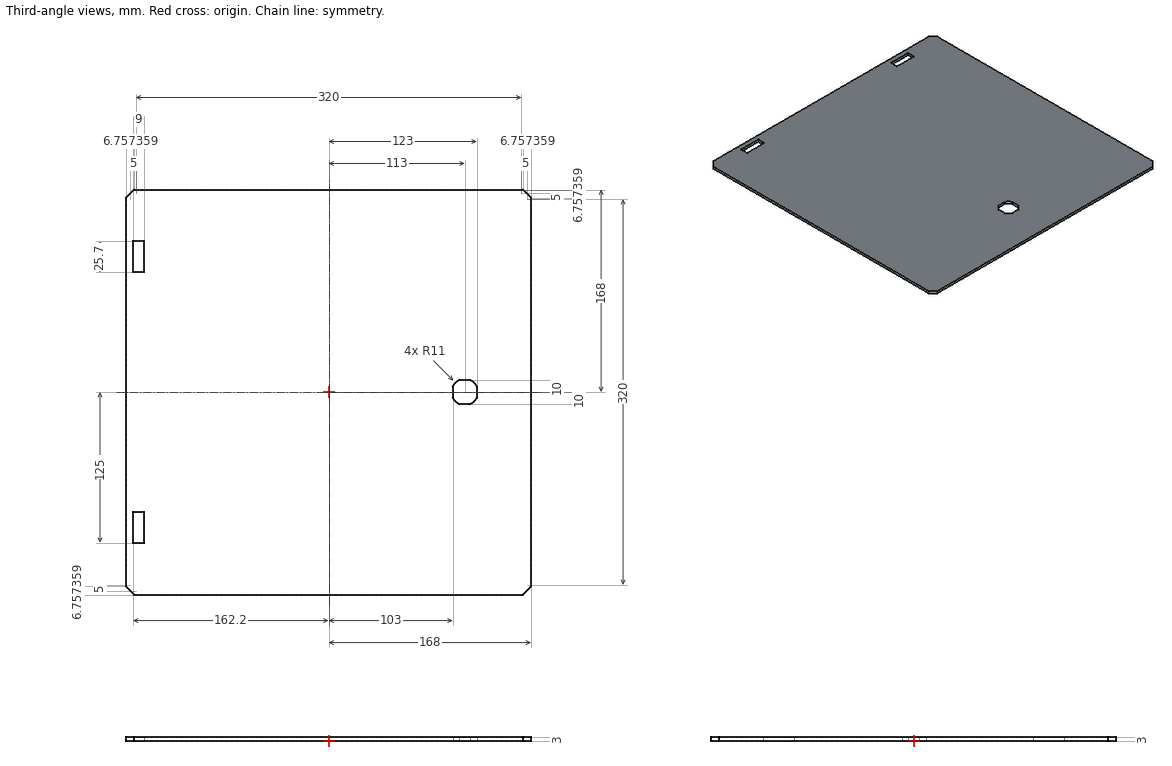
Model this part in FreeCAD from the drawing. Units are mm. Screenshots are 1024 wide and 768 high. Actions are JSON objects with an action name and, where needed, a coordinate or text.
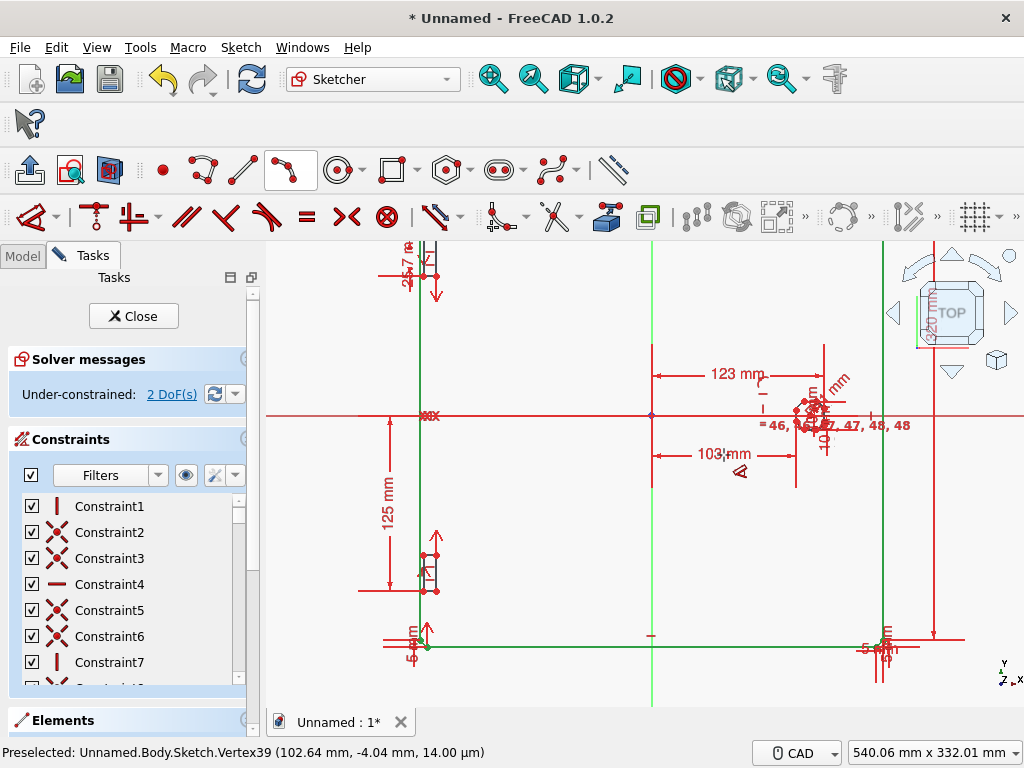
{"action": "left_click", "coordinate": [811, 416]}
{"action": "left_click", "coordinate": [731, 498]}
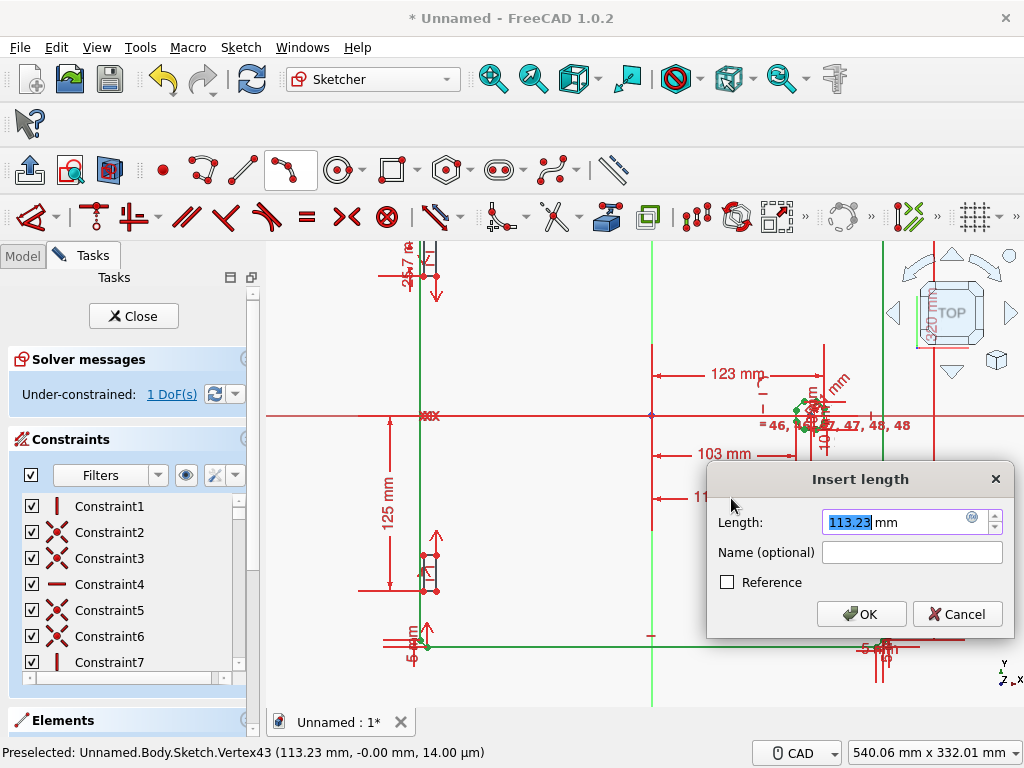
{"action": "type", "text": "113"}
{"action": "key", "text": "Return"}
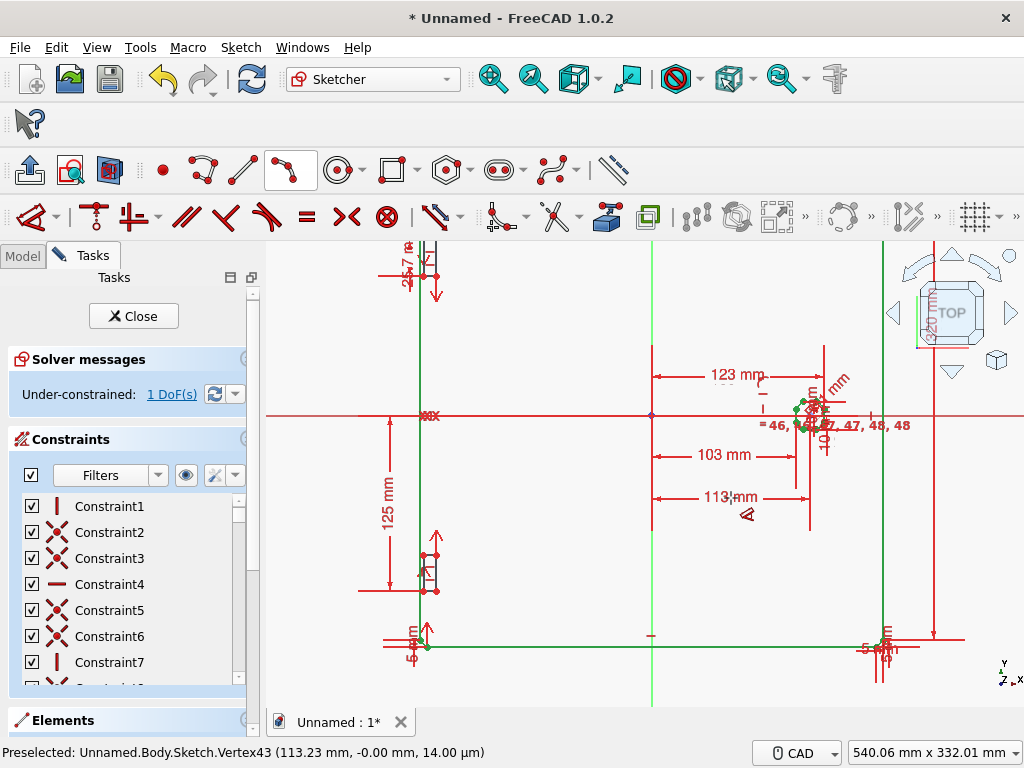
{"action": "left_click", "coordinate": [424, 555]}
{"action": "left_click", "coordinate": [538, 589]}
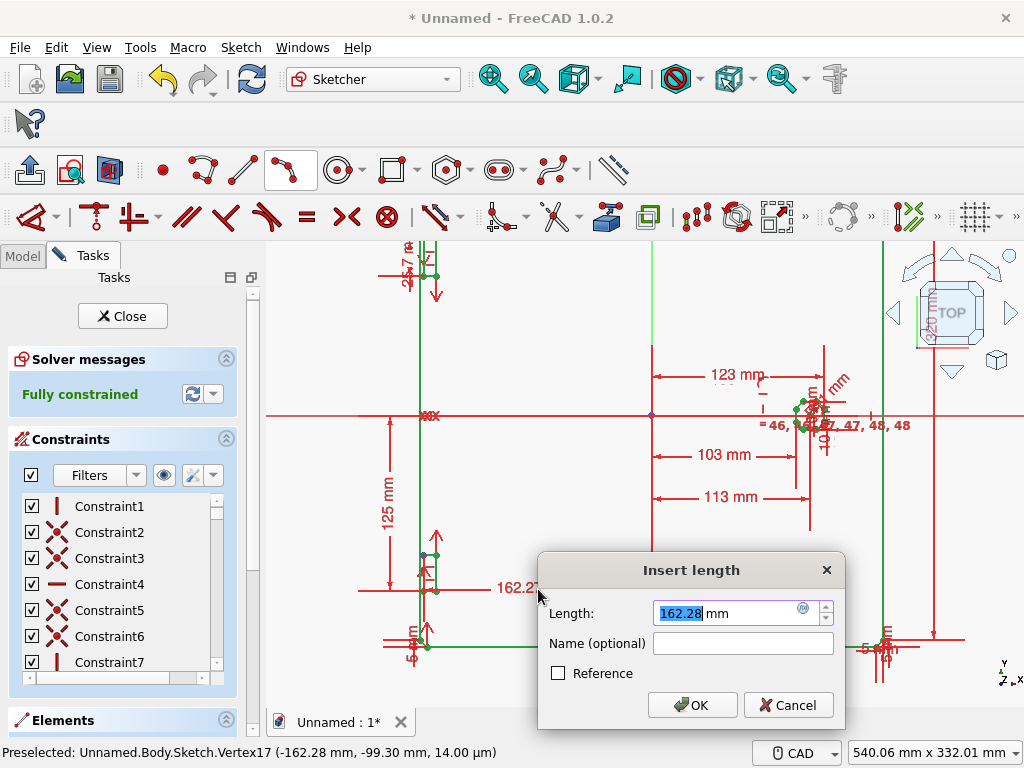
{"action": "type", "text": "162.2"}
{"action": "key", "text": "Return"}
{"action": "key", "text": "Escape"}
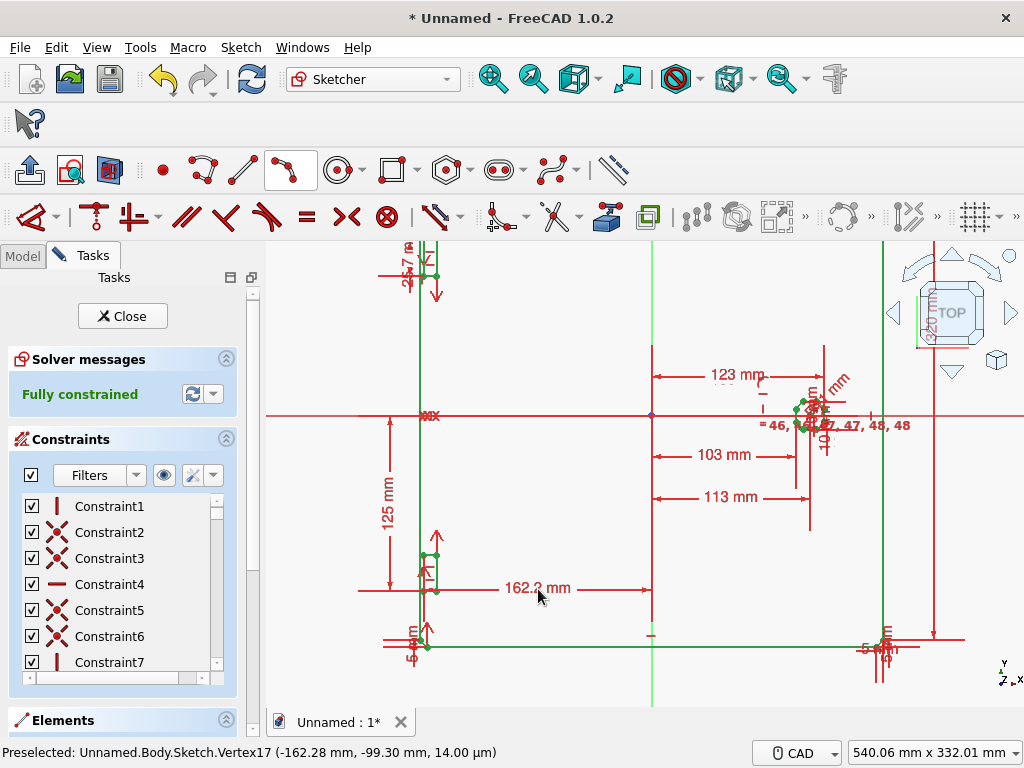
{"action": "left_click", "coordinate": [123, 316]}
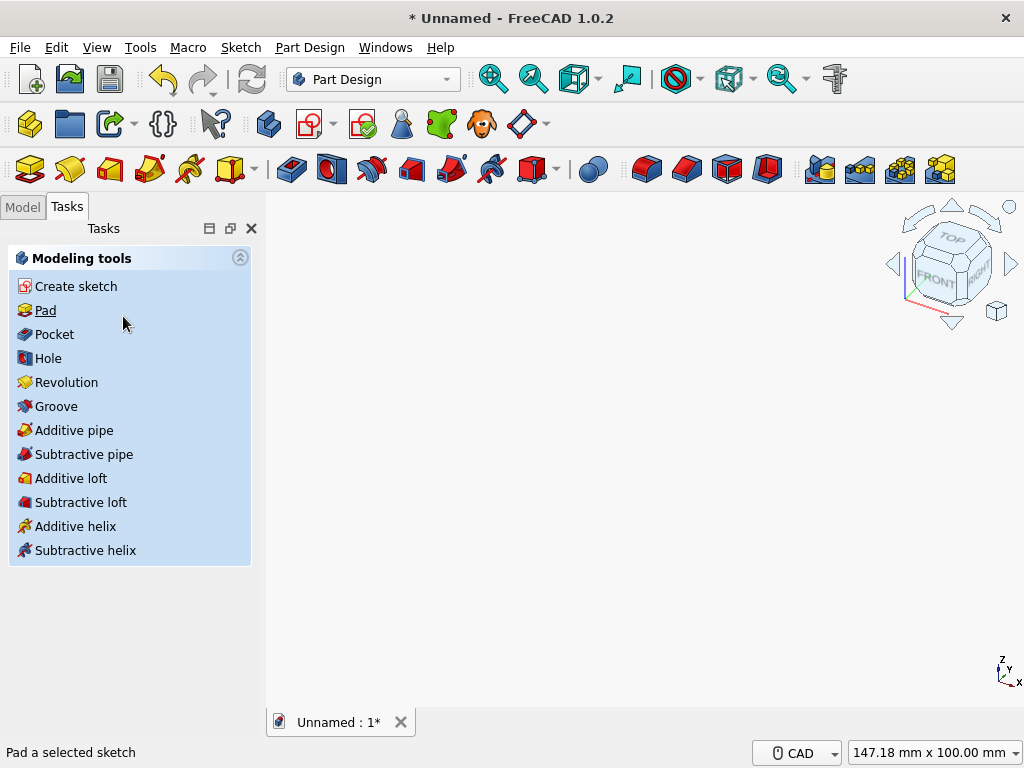
{"action": "left_click", "coordinate": [30, 170]}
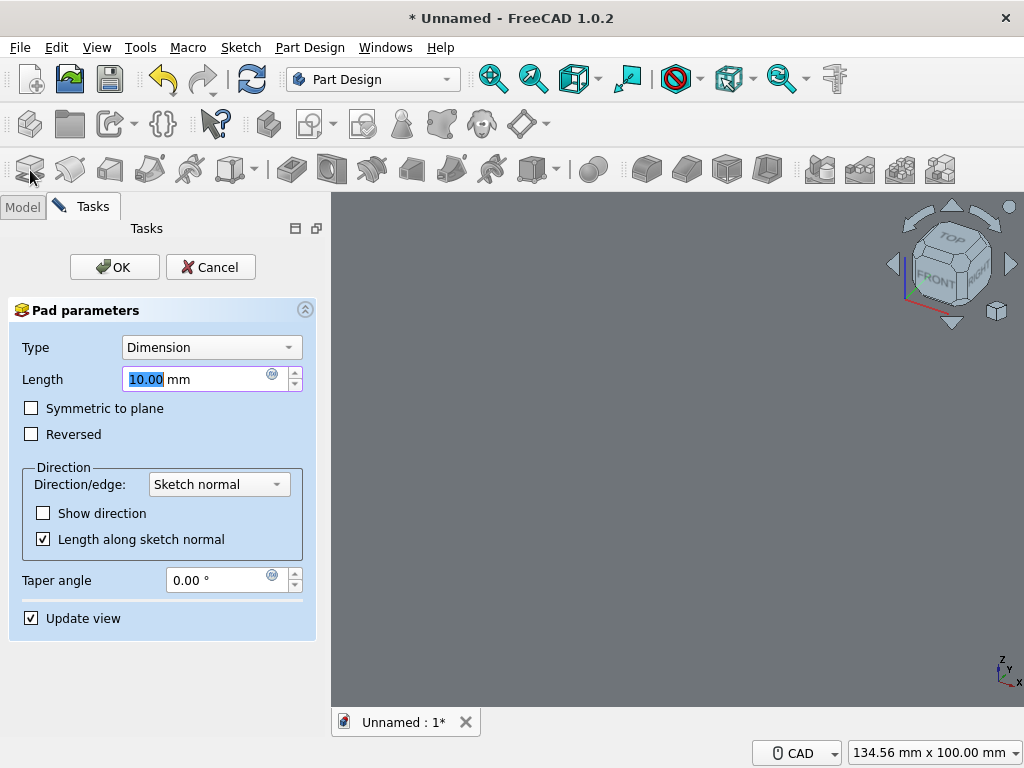
{"action": "type", "text": "3"}
{"action": "key", "text": "Tab"}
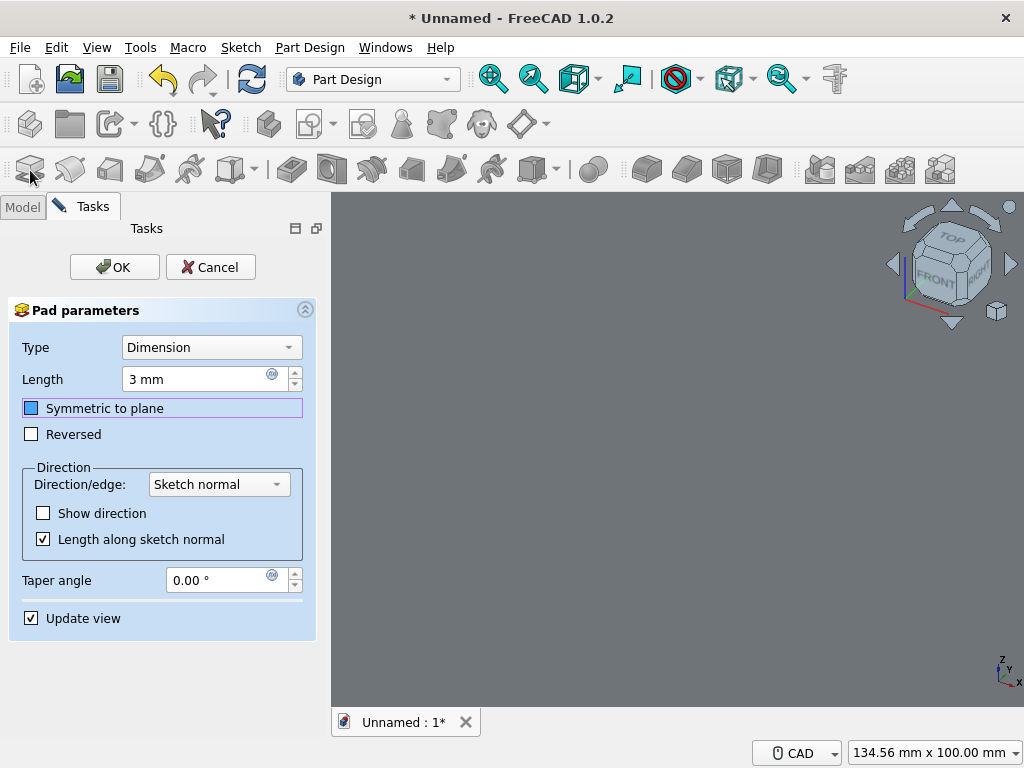
{"action": "left_click", "coordinate": [115, 267]}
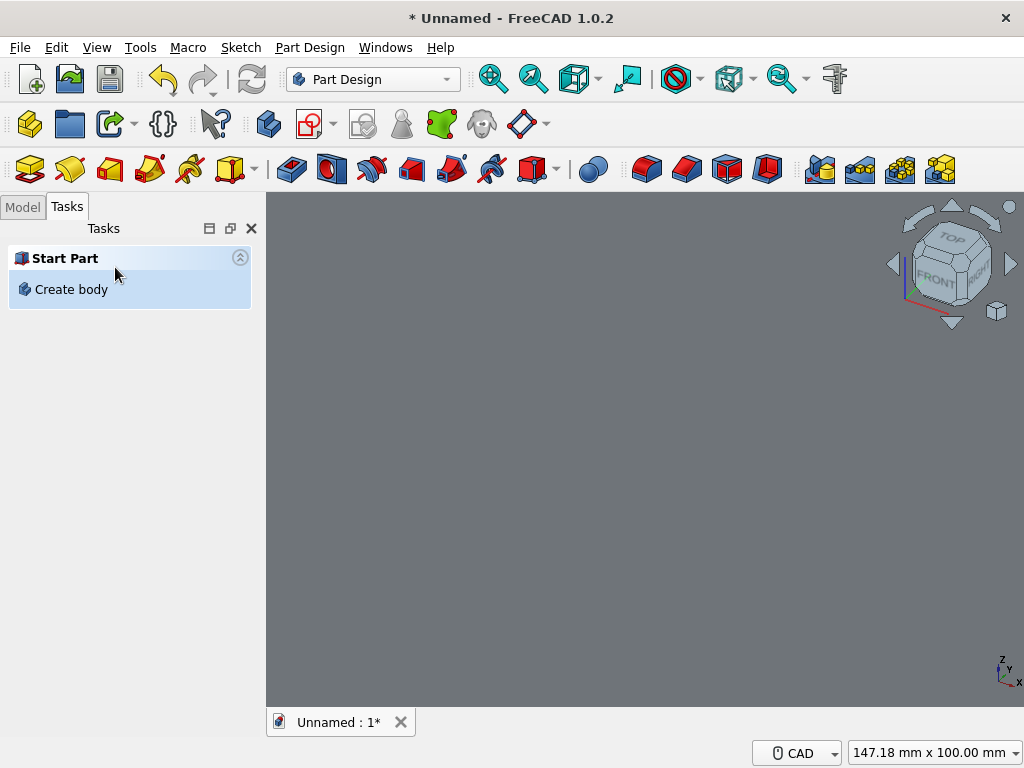
{"action": "left_click", "coordinate": [494, 80]}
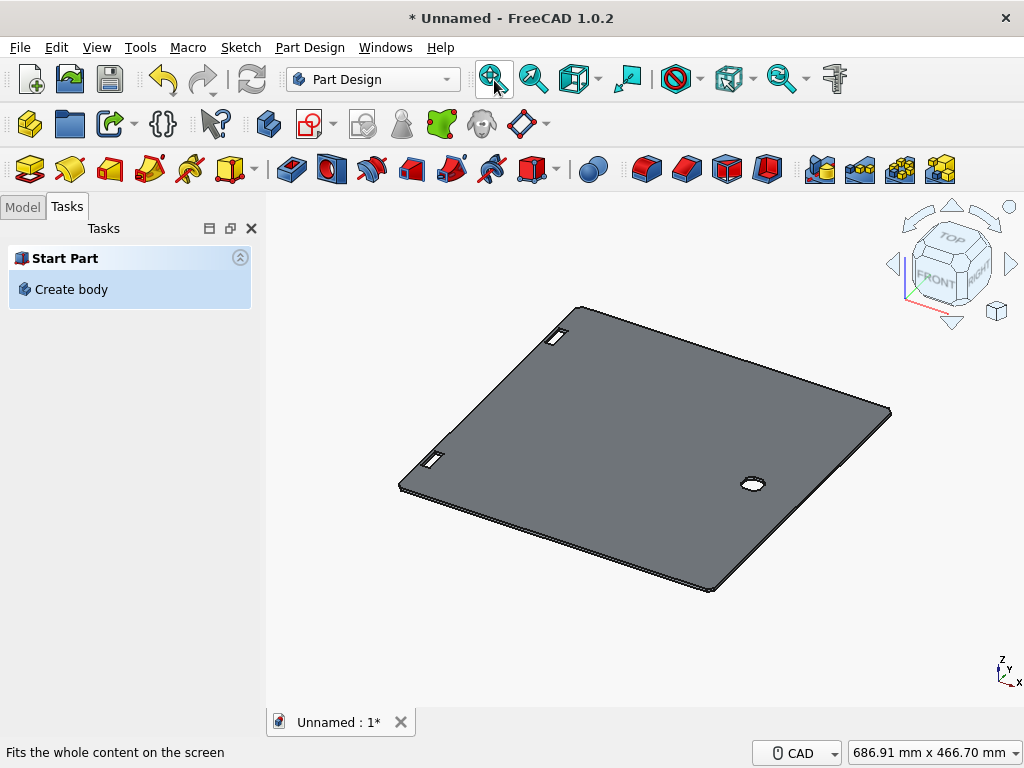
{"action": "left_click", "coordinate": [626, 406]}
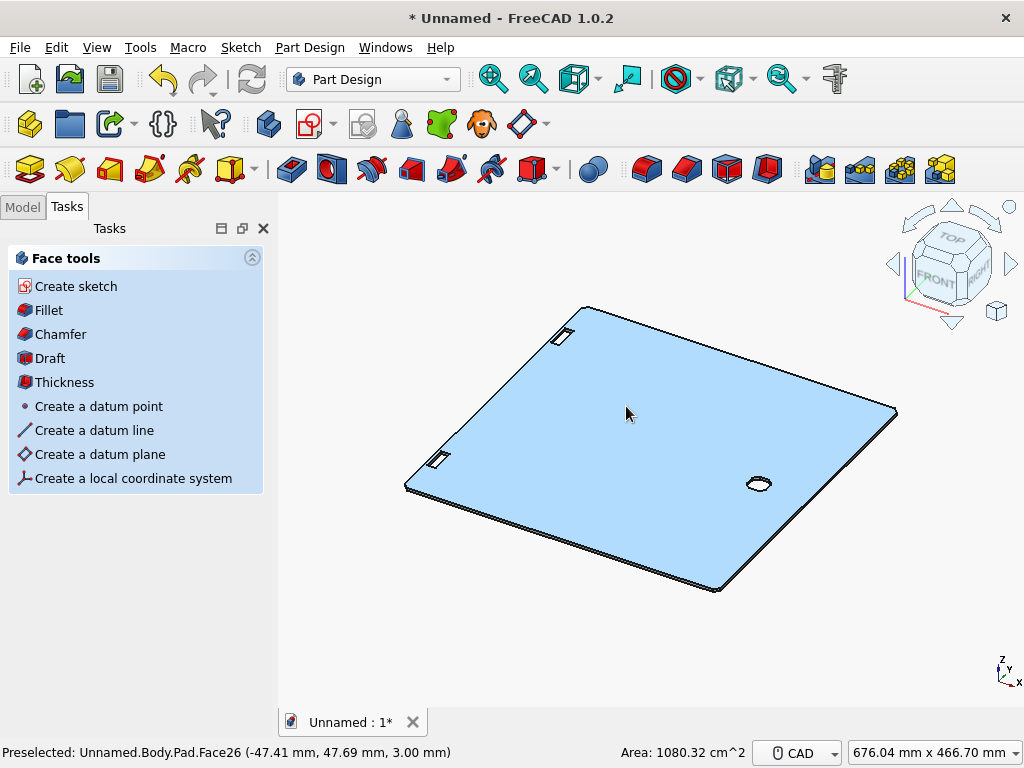
{"action": "left_click", "coordinate": [310, 124]}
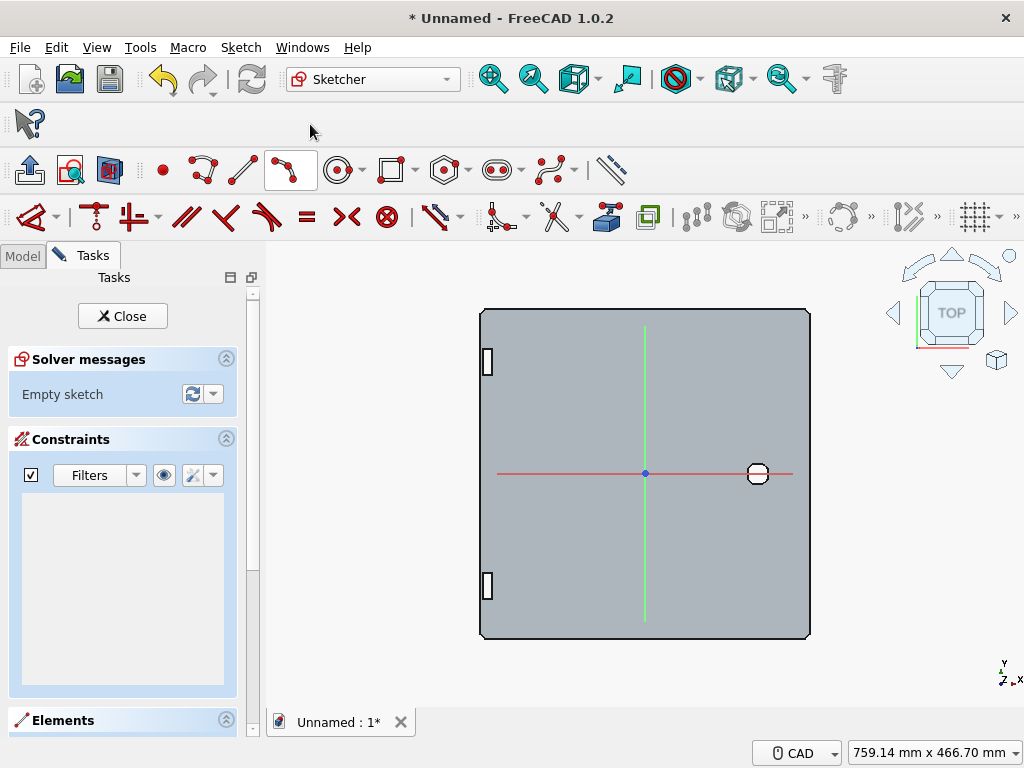
{"action": "left_click", "coordinate": [204, 170]}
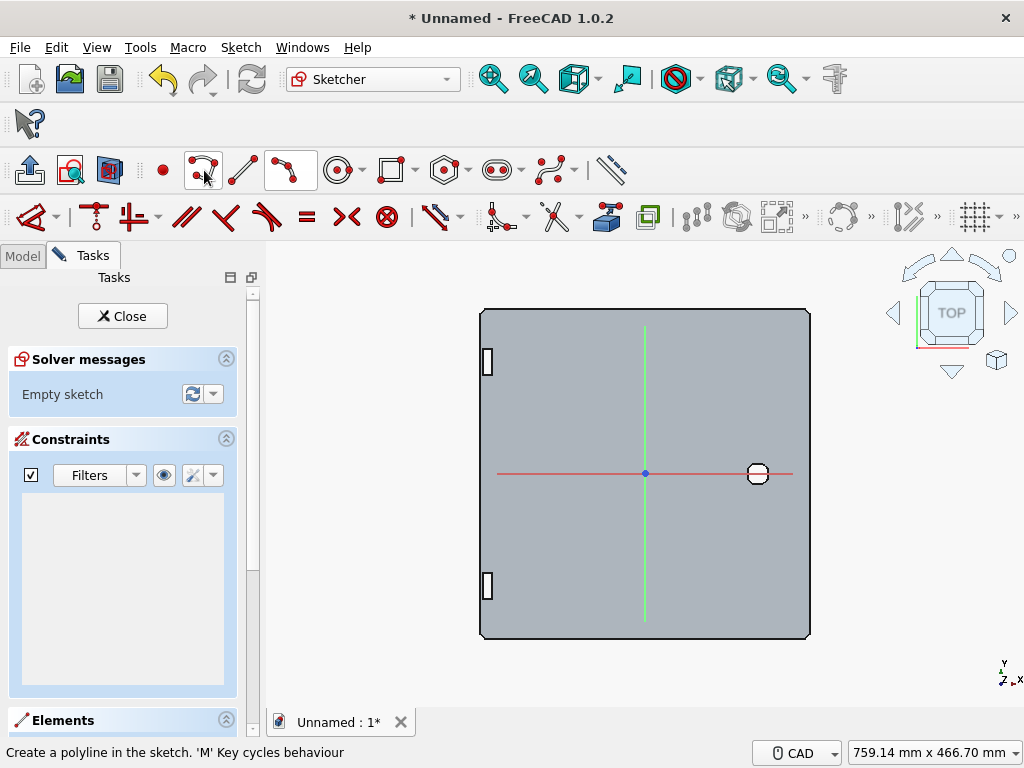
{"action": "left_click", "coordinate": [813, 635]}
{"action": "left_click", "coordinate": [813, 313]}